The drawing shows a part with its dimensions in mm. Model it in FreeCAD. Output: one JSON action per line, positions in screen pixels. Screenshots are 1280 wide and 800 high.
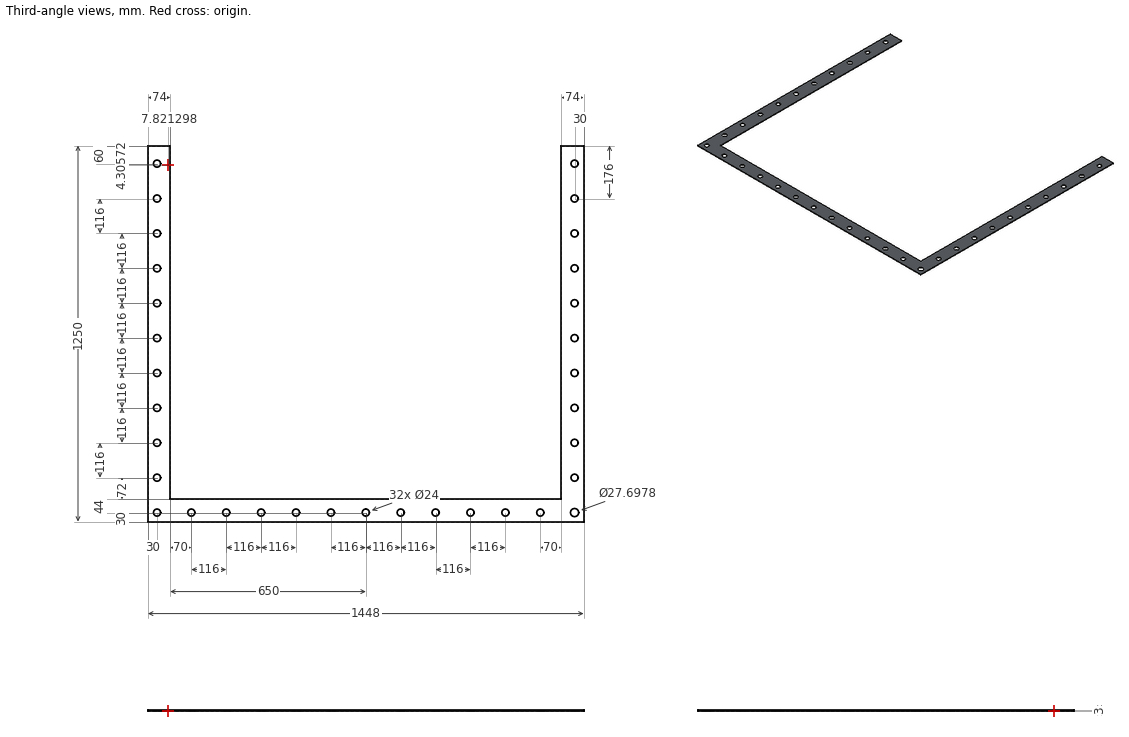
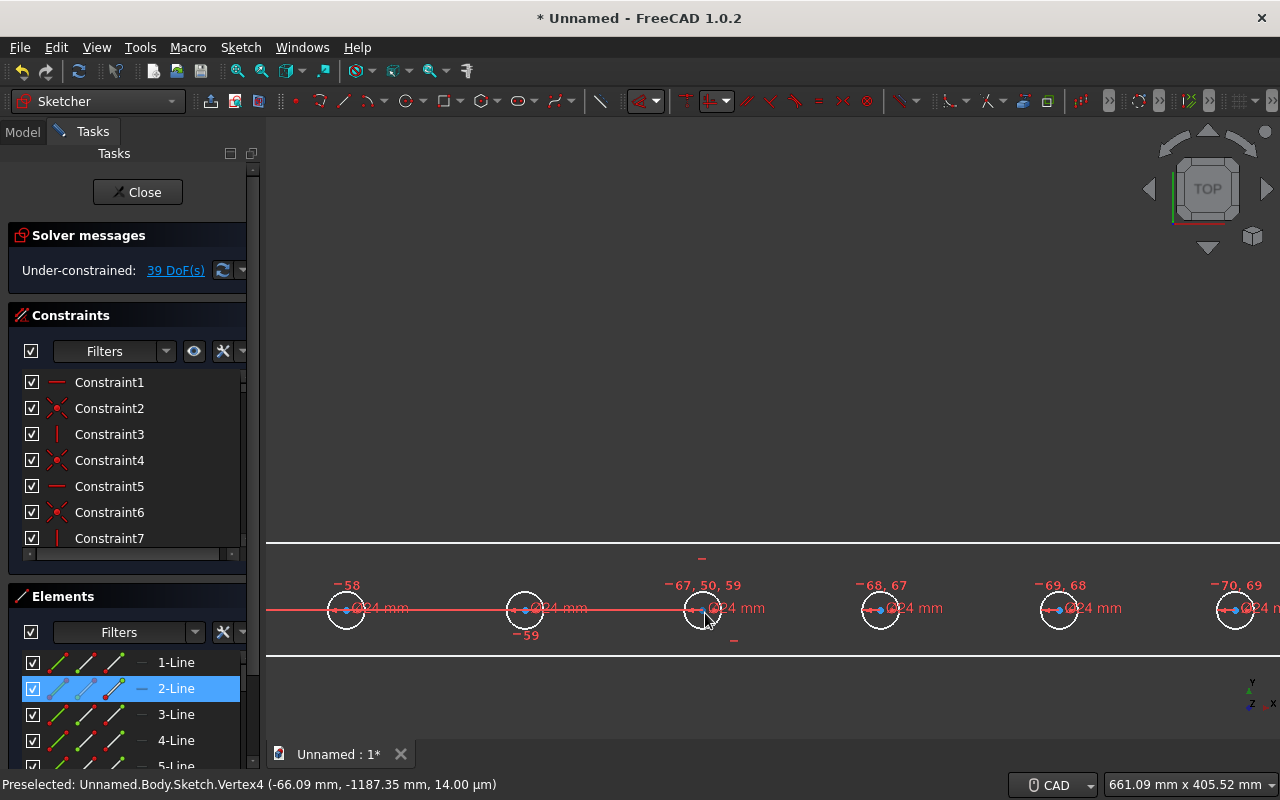
{"action": "left_click", "coordinate": [703, 610]}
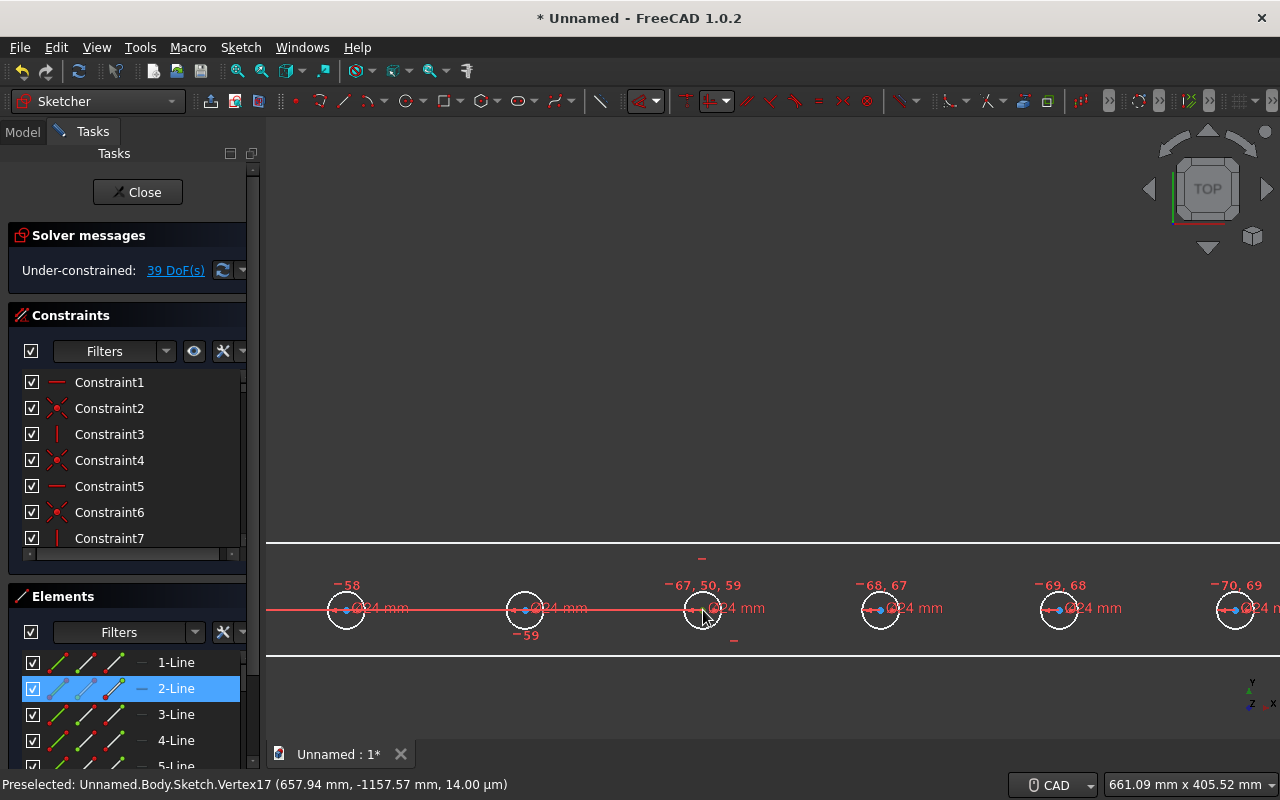
{"action": "left_click", "coordinate": [658, 102]}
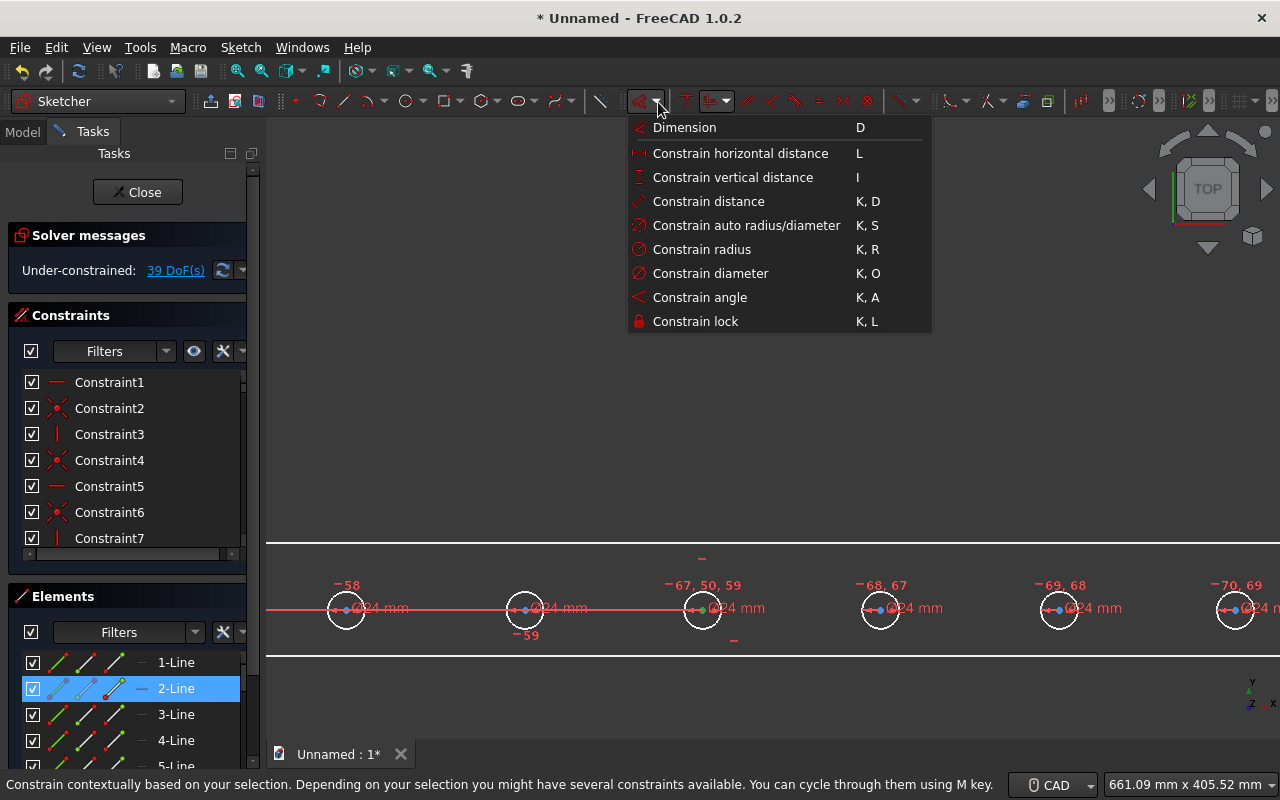
{"action": "left_click", "coordinate": [780, 177]}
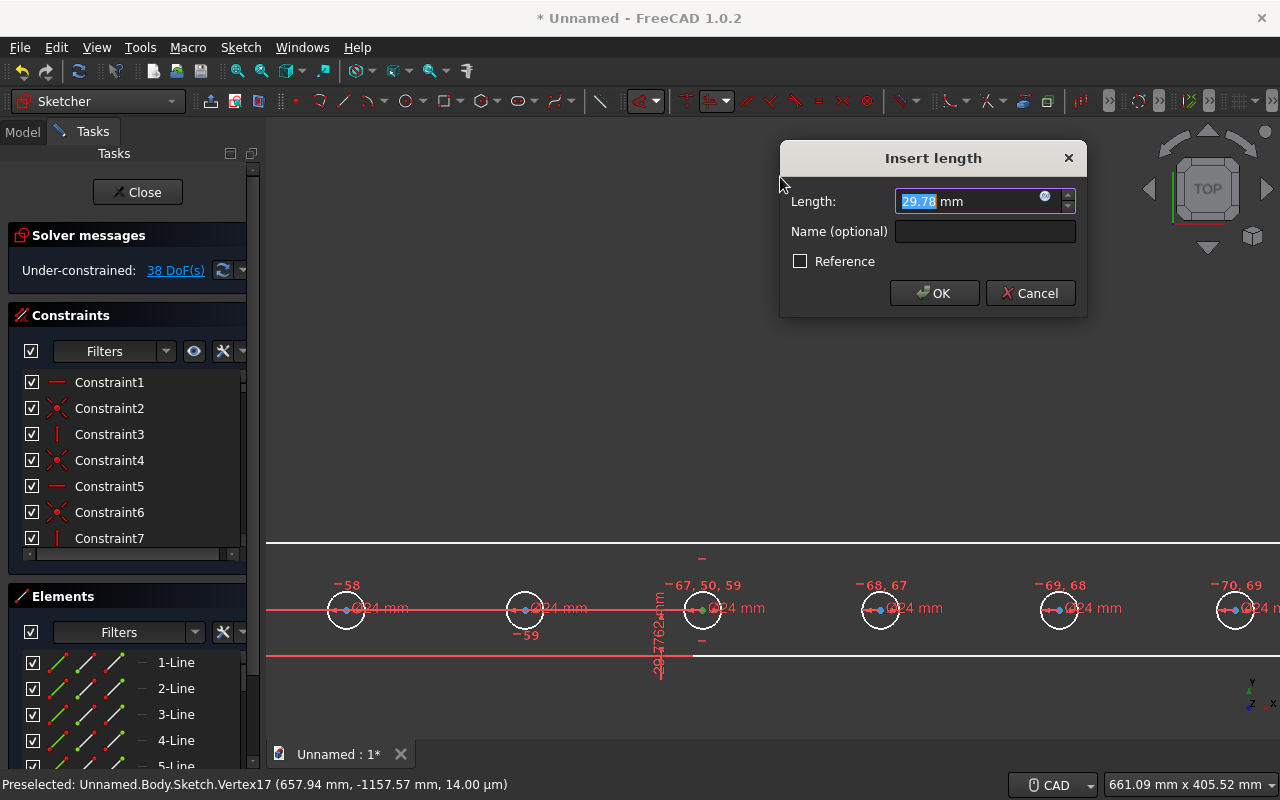
{"action": "type", "text": "30"}
{"action": "key", "text": "Return"}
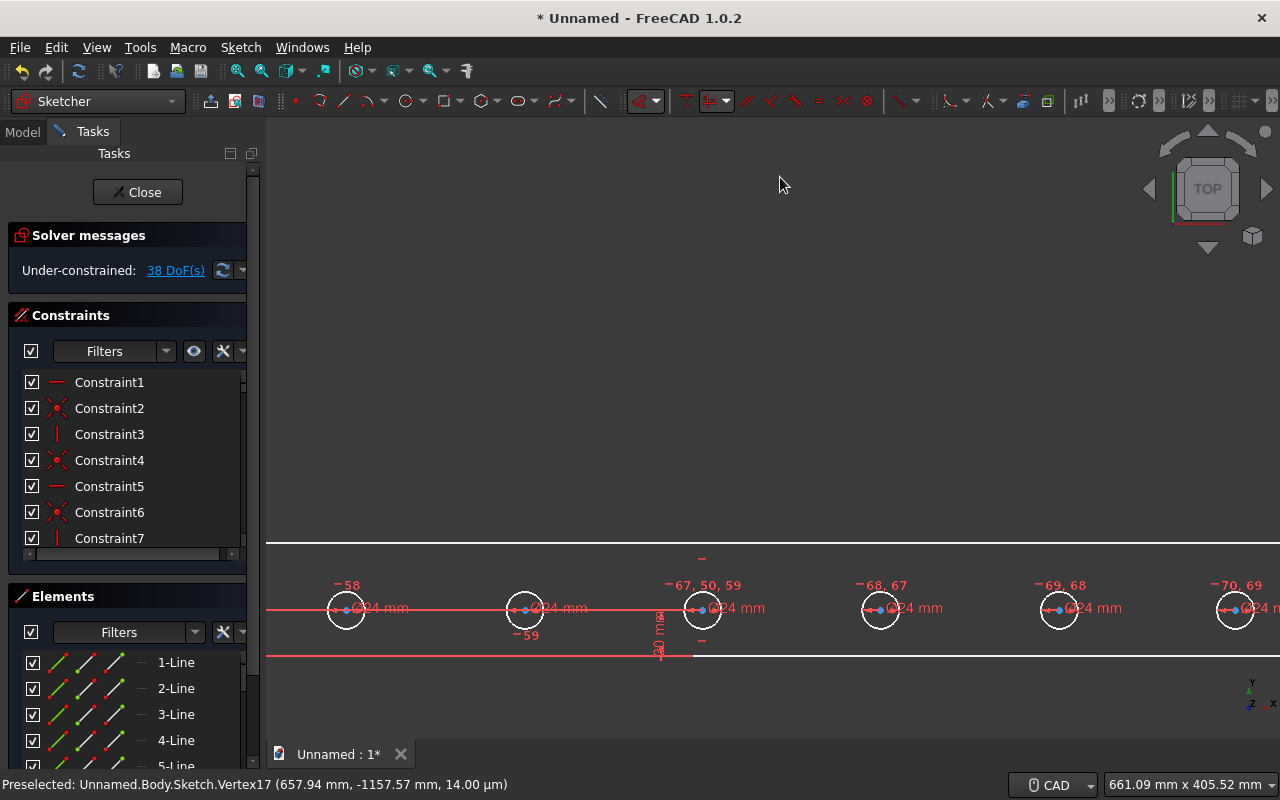
{"action": "scroll", "coordinate": [705, 613], "scroll_direction": "down", "scroll_amount": 8}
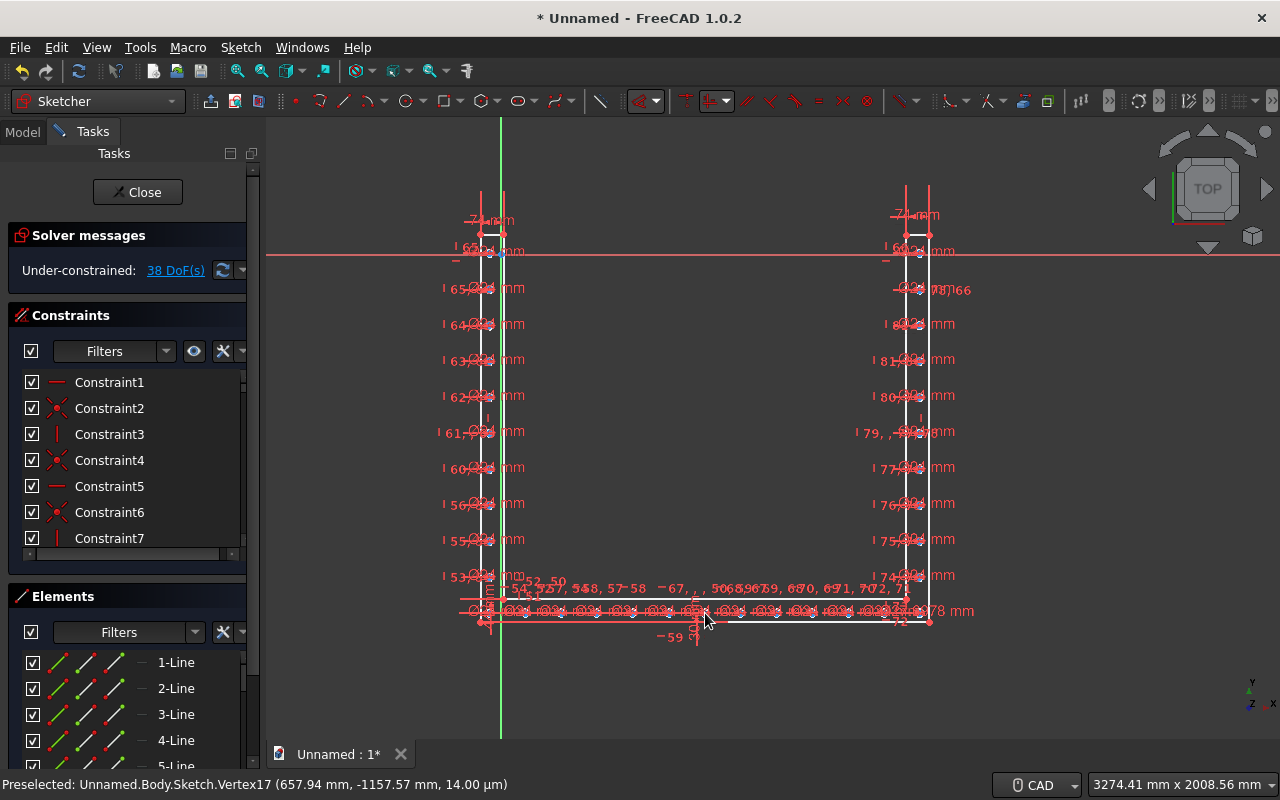
{"action": "scroll", "coordinate": [481, 622], "scroll_direction": "up", "scroll_amount": 8}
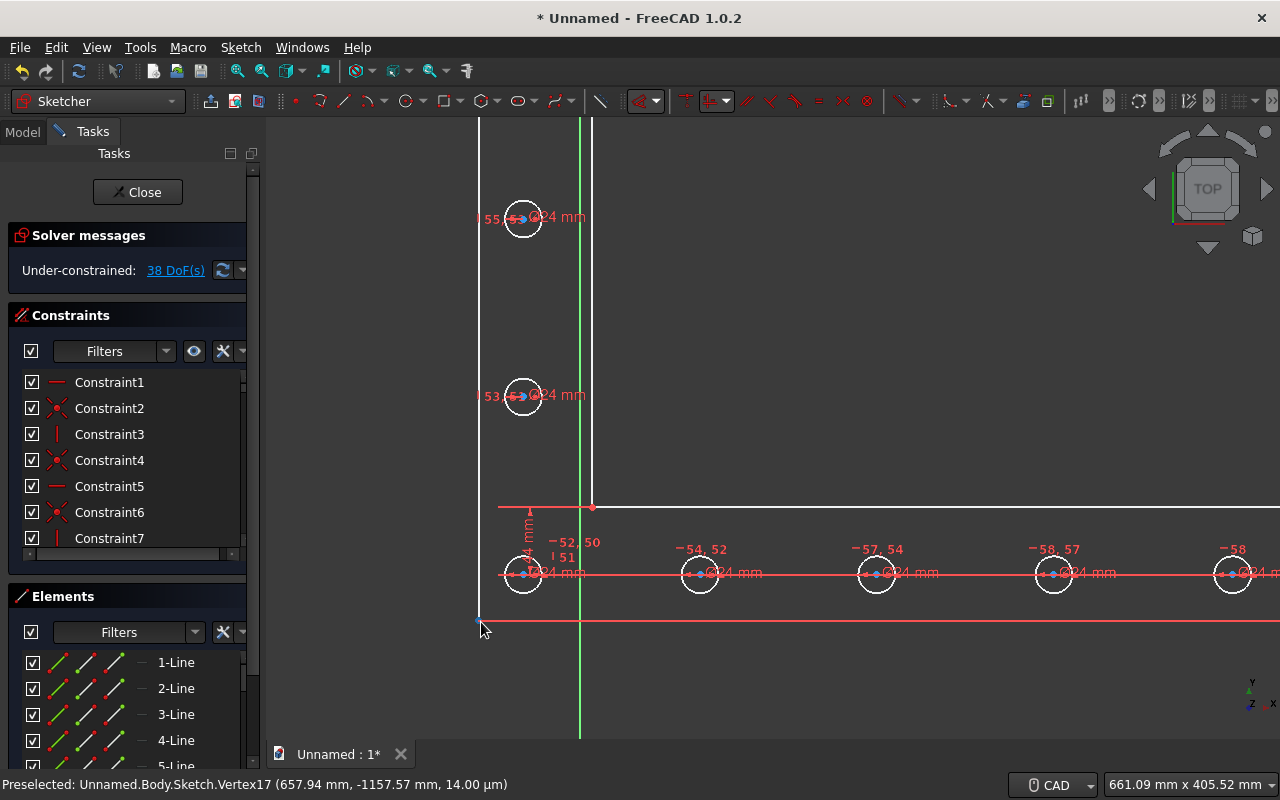
{"action": "left_click", "coordinate": [479, 621]}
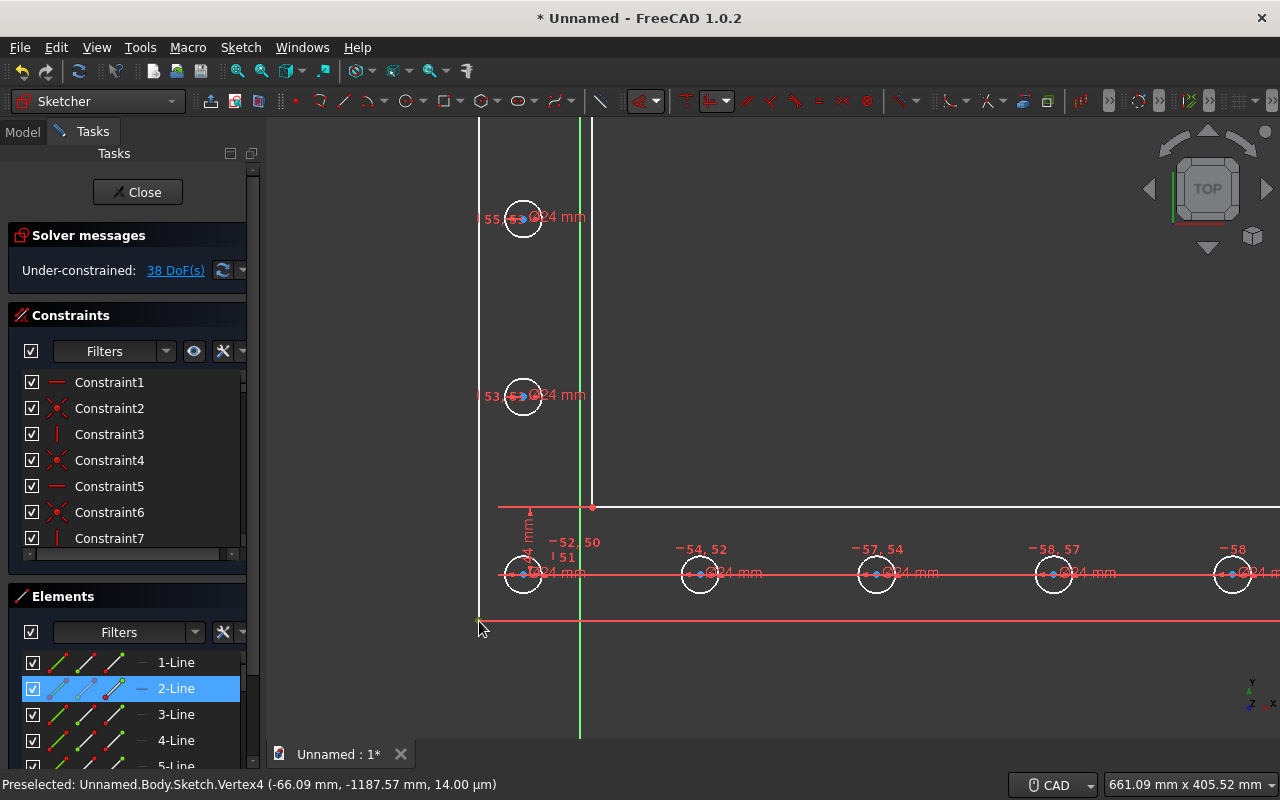
{"action": "left_click", "coordinate": [523, 575]}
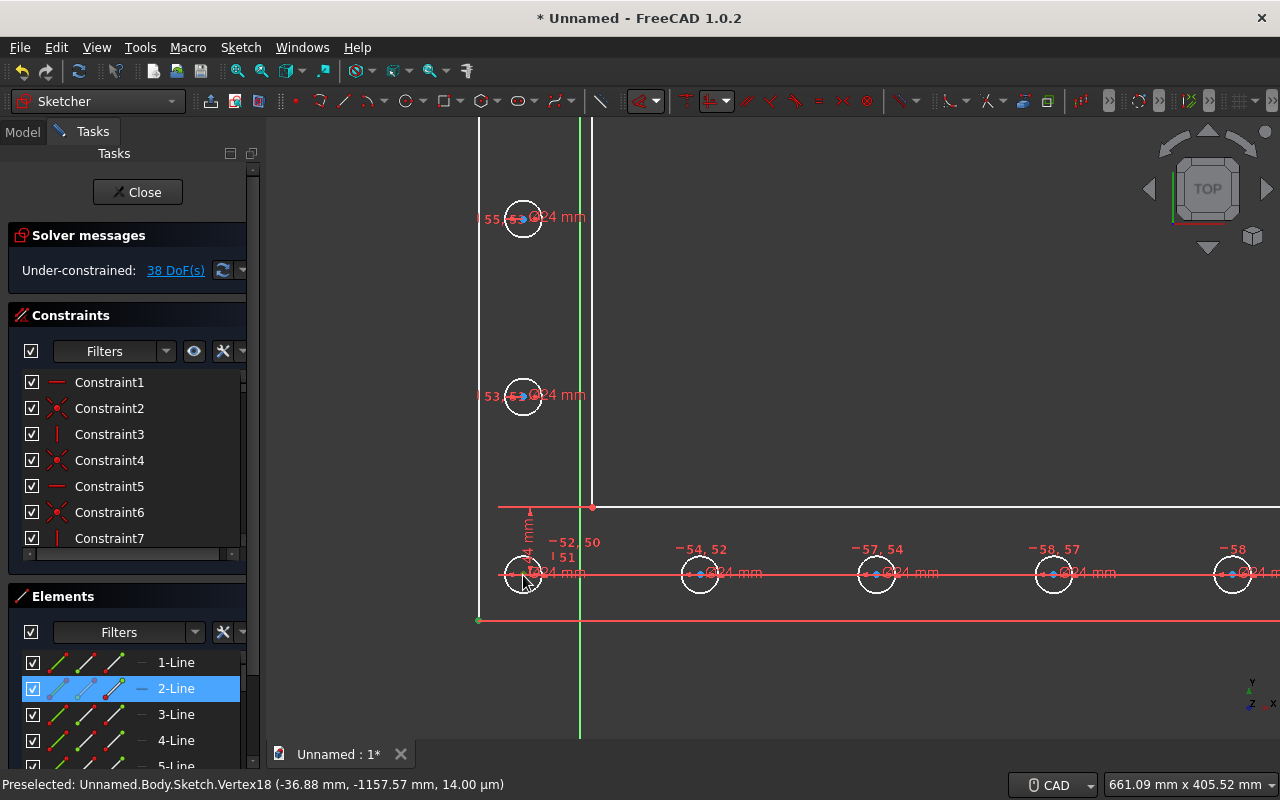
{"action": "left_click", "coordinate": [658, 102]}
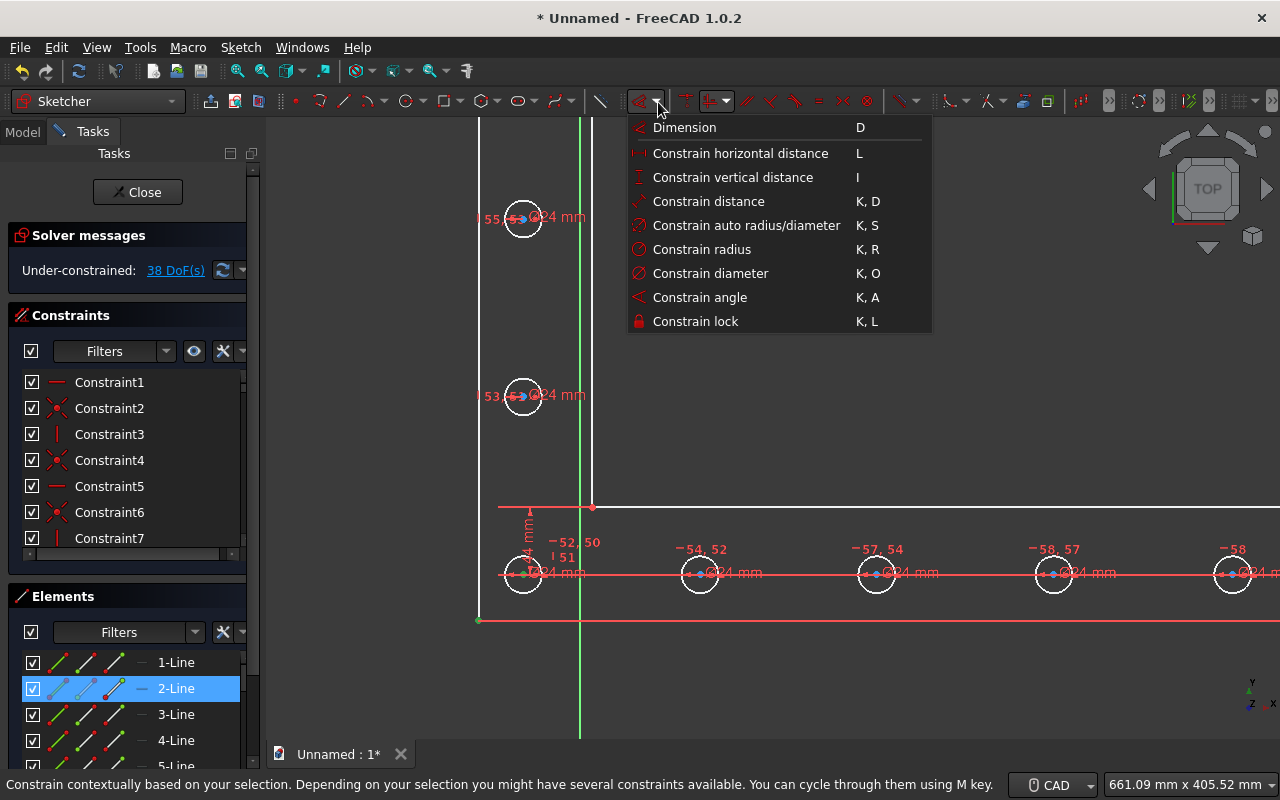
{"action": "left_click", "coordinate": [780, 153]}